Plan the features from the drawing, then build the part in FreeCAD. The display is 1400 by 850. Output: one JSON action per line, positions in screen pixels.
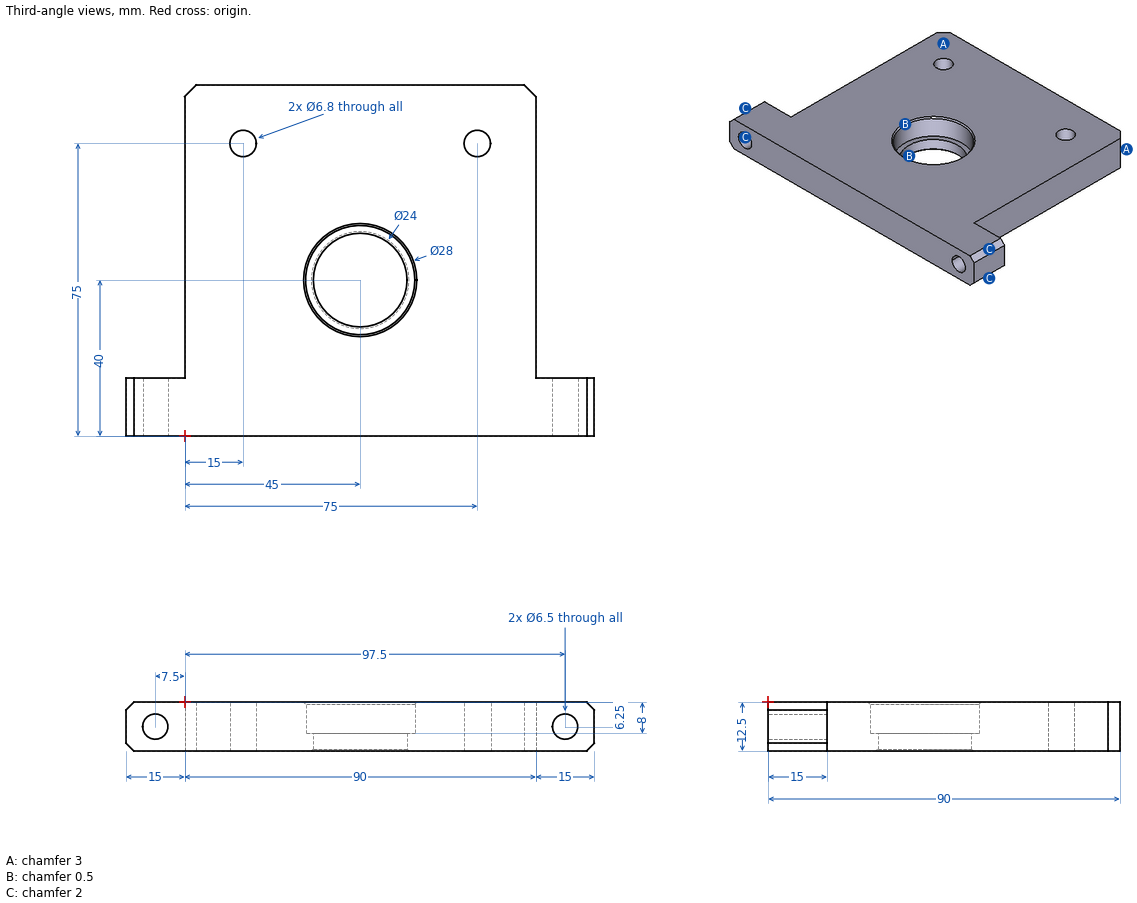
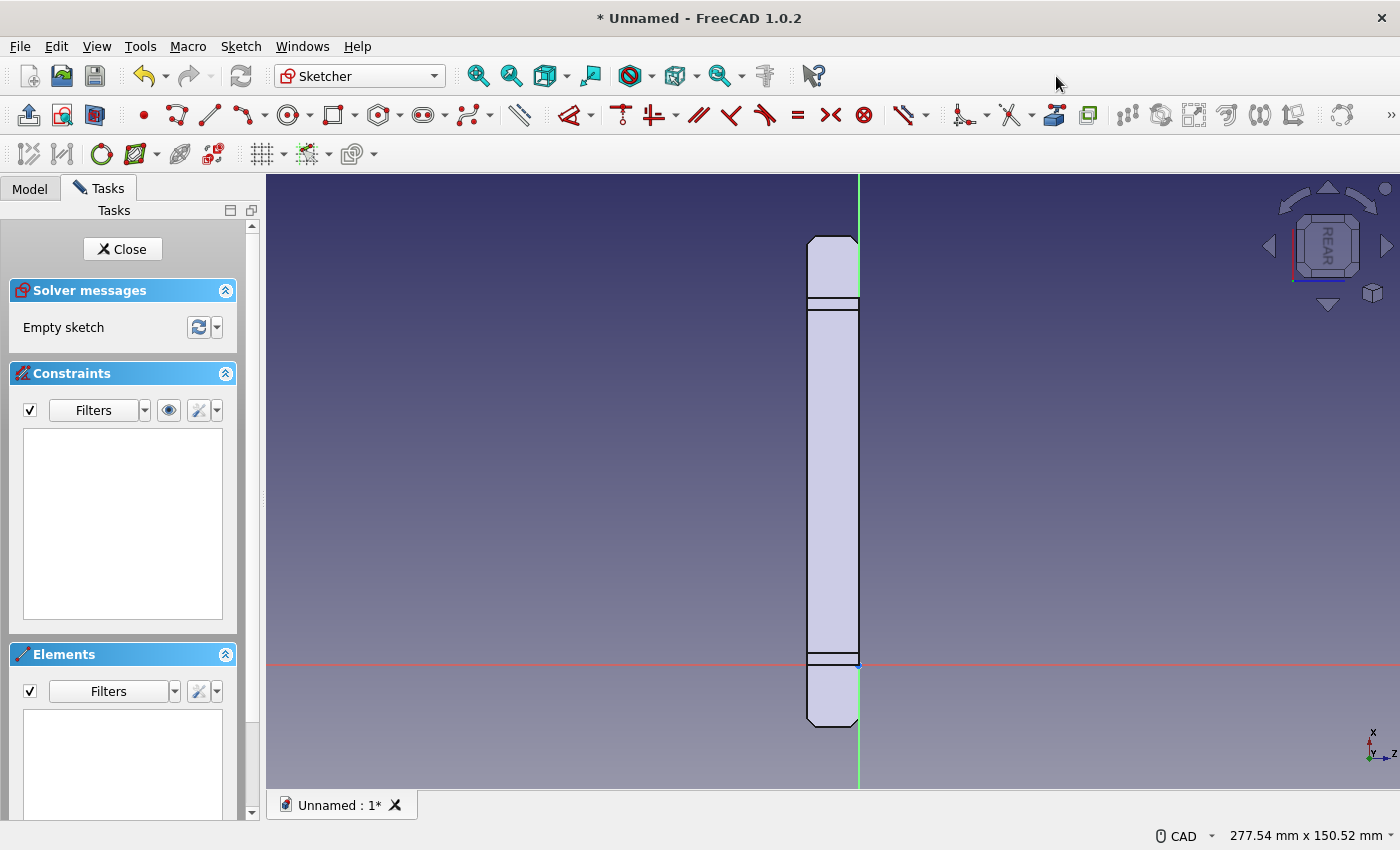
{"action": "left_click", "coordinate": [95, 116]}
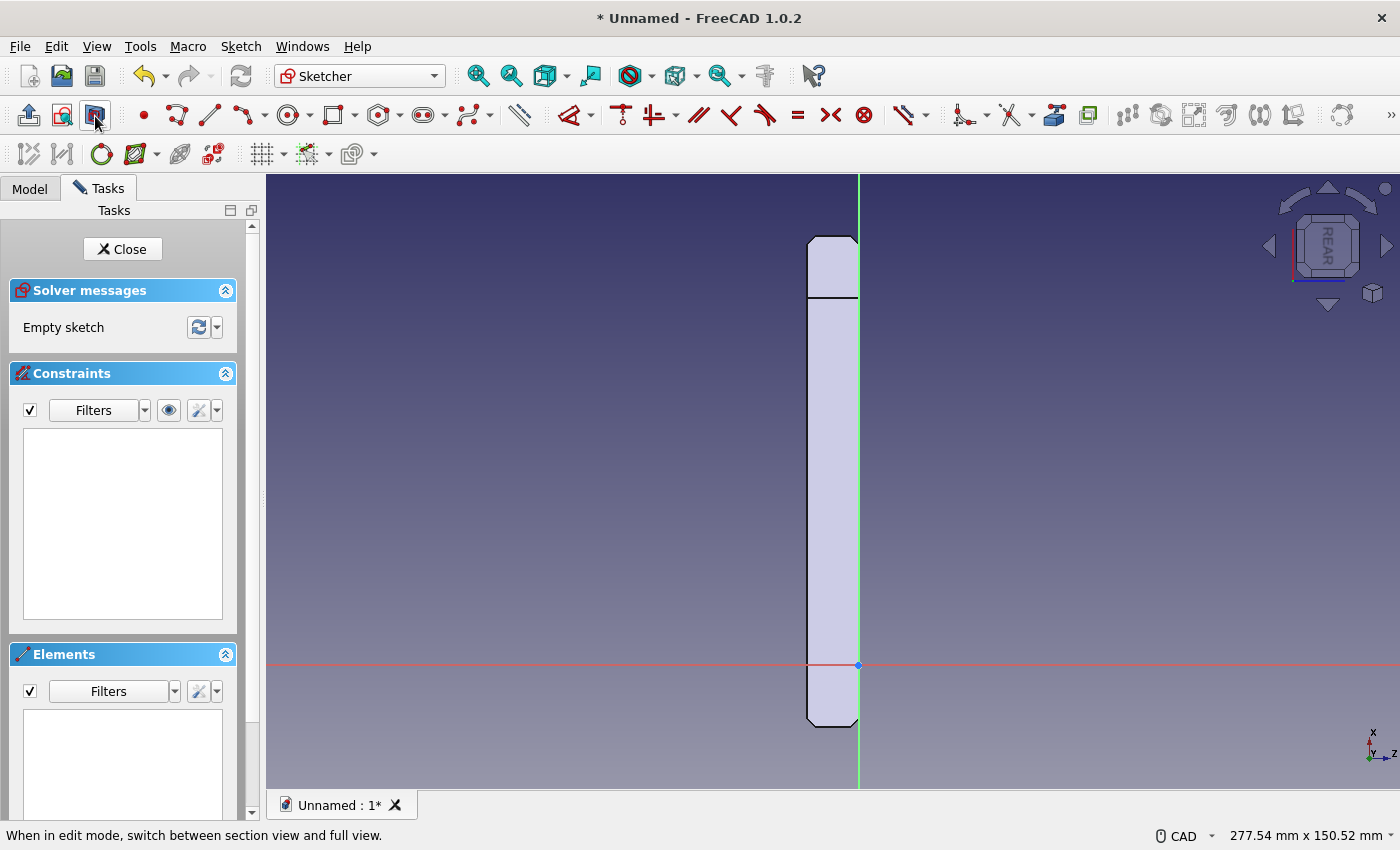
{"action": "left_click", "coordinate": [288, 116]}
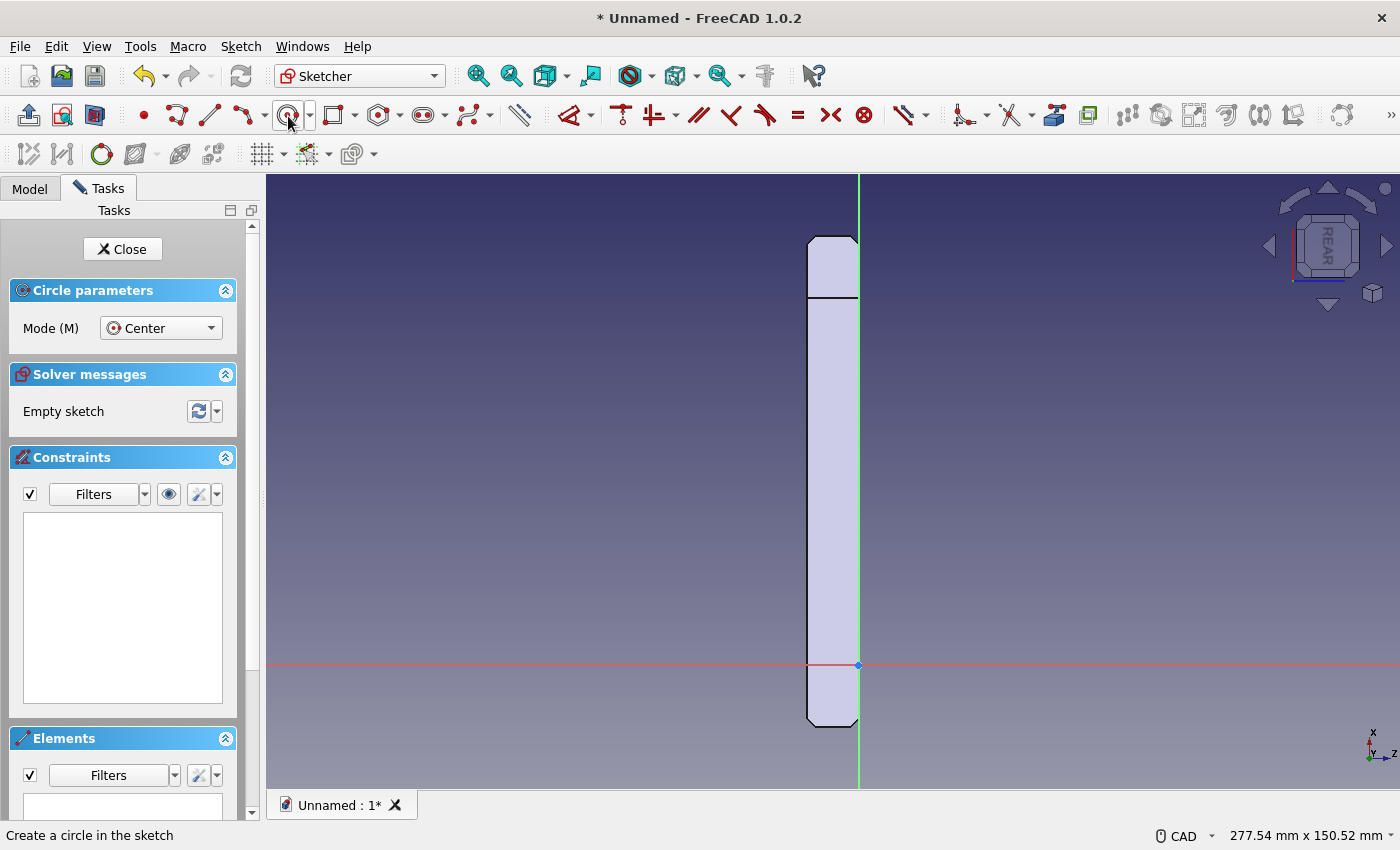
{"action": "scroll", "coordinate": [833, 267], "scroll_direction": "up", "scroll_amount": 3}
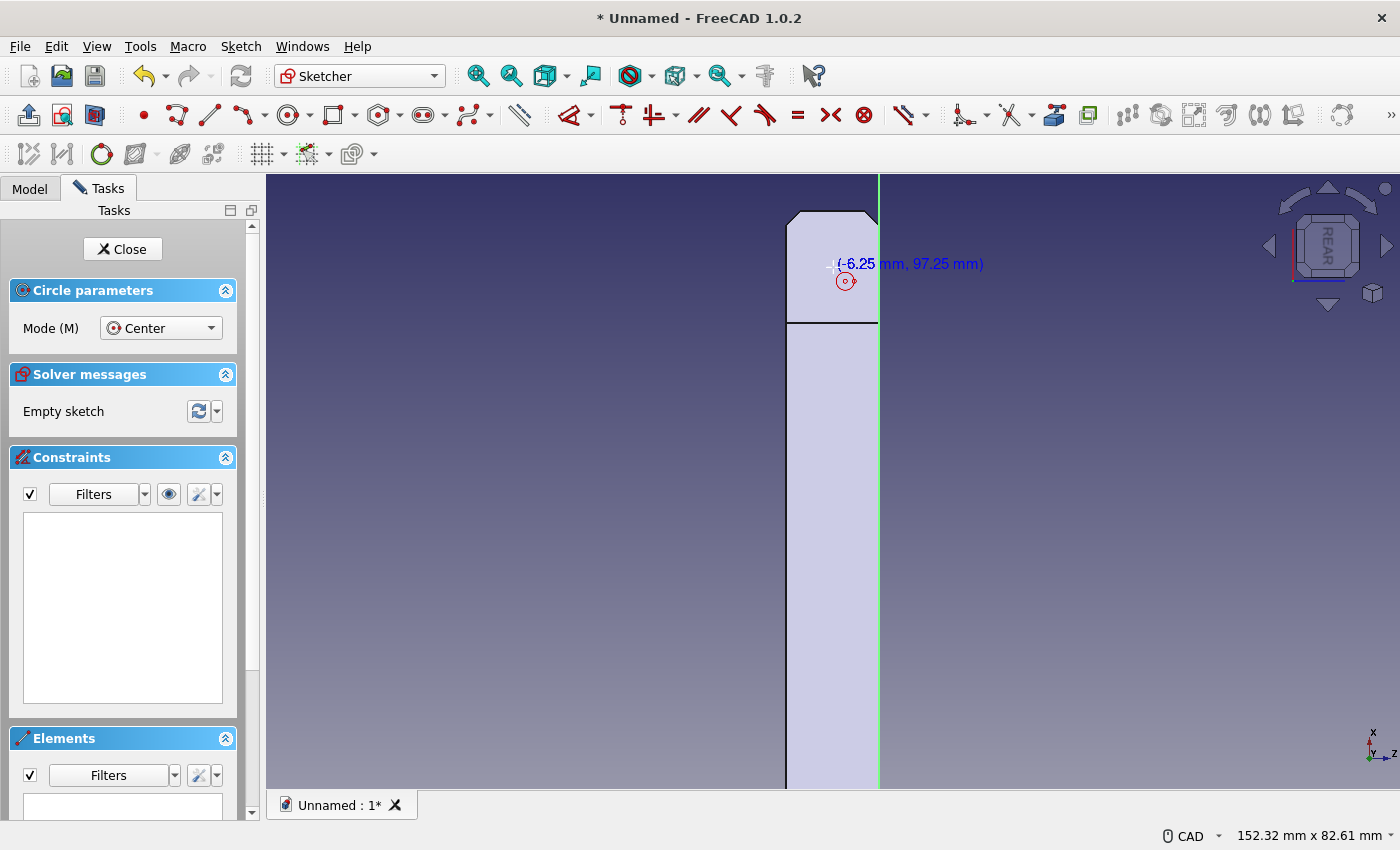
{"action": "left_click", "coordinate": [833, 267]}
{"action": "left_click", "coordinate": [850, 250]}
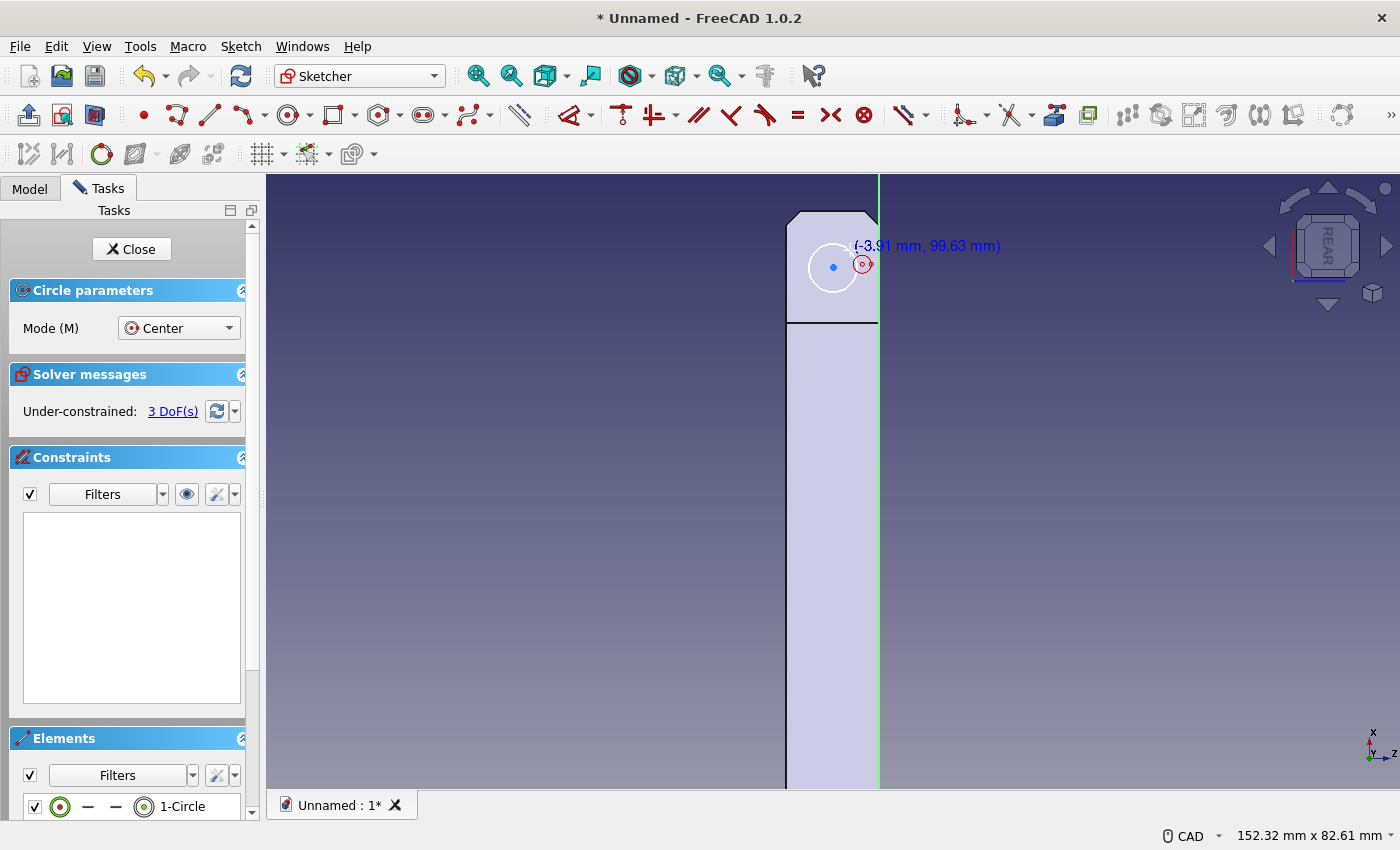
{"action": "scroll", "coordinate": [700, 338], "scroll_direction": "down", "scroll_amount": 4}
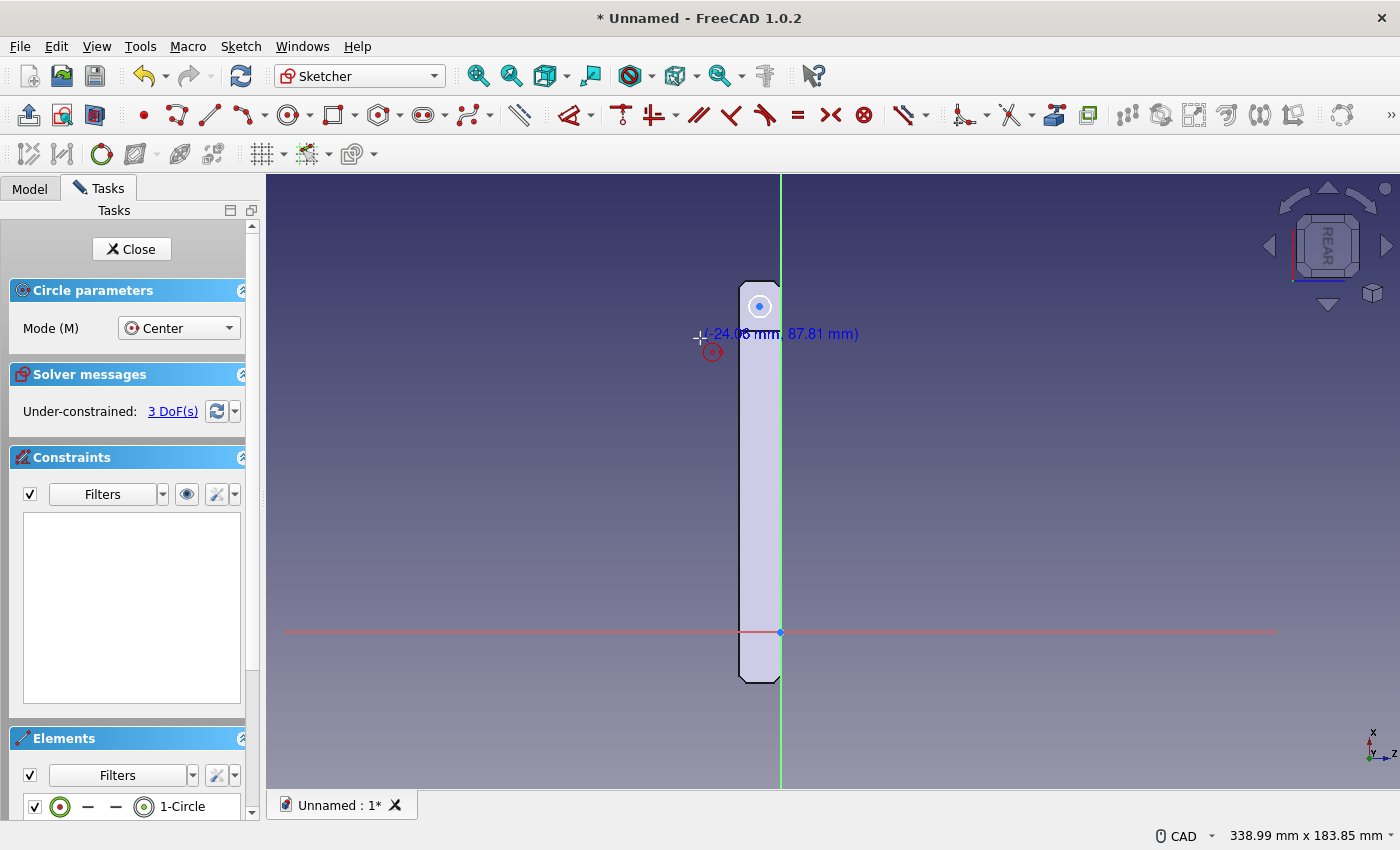
{"action": "scroll", "coordinate": [760, 657], "scroll_direction": "up", "scroll_amount": 4}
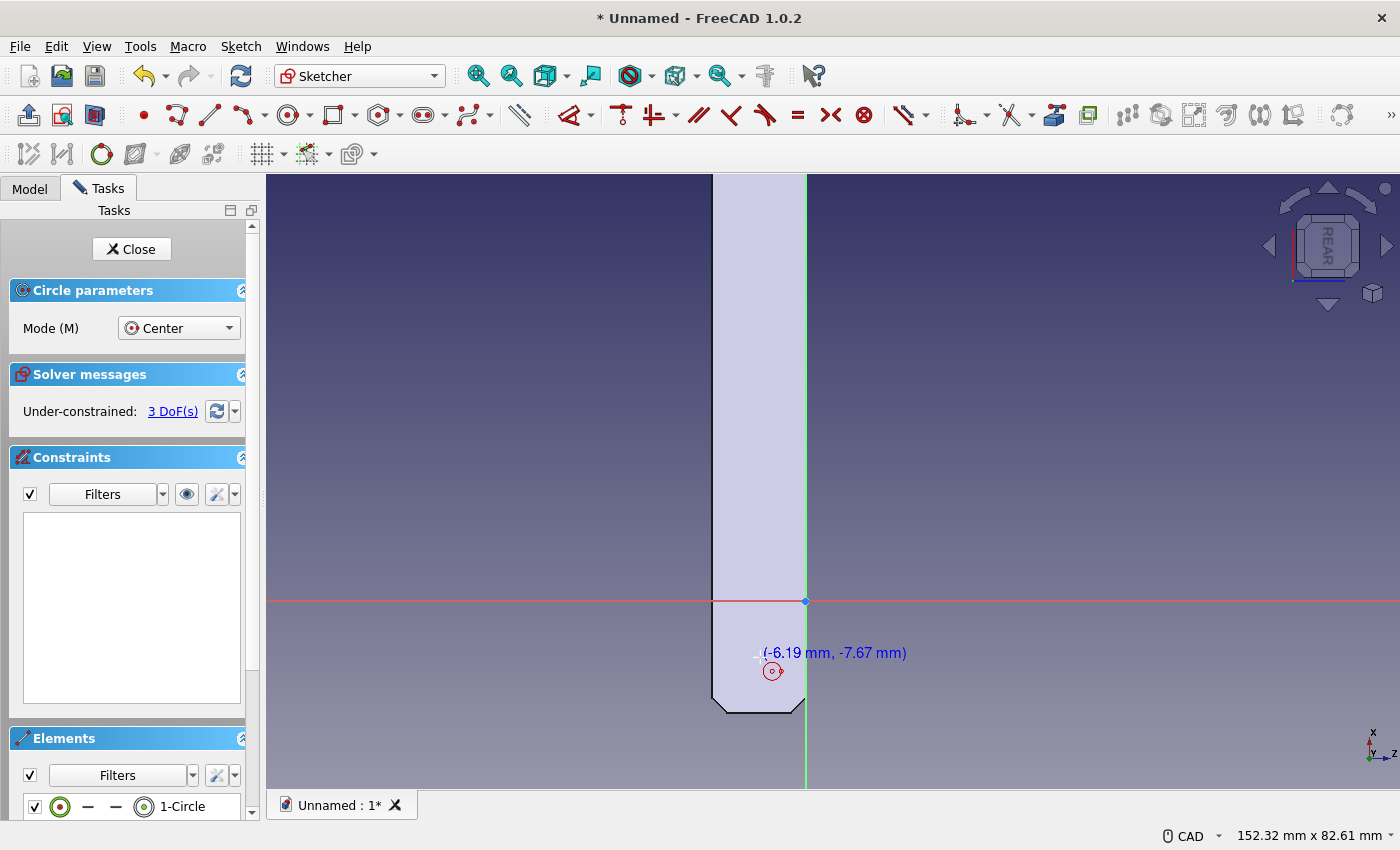
{"action": "left_click", "coordinate": [759, 657]}
{"action": "left_click", "coordinate": [776, 640]}
{"action": "key", "text": "Escape"}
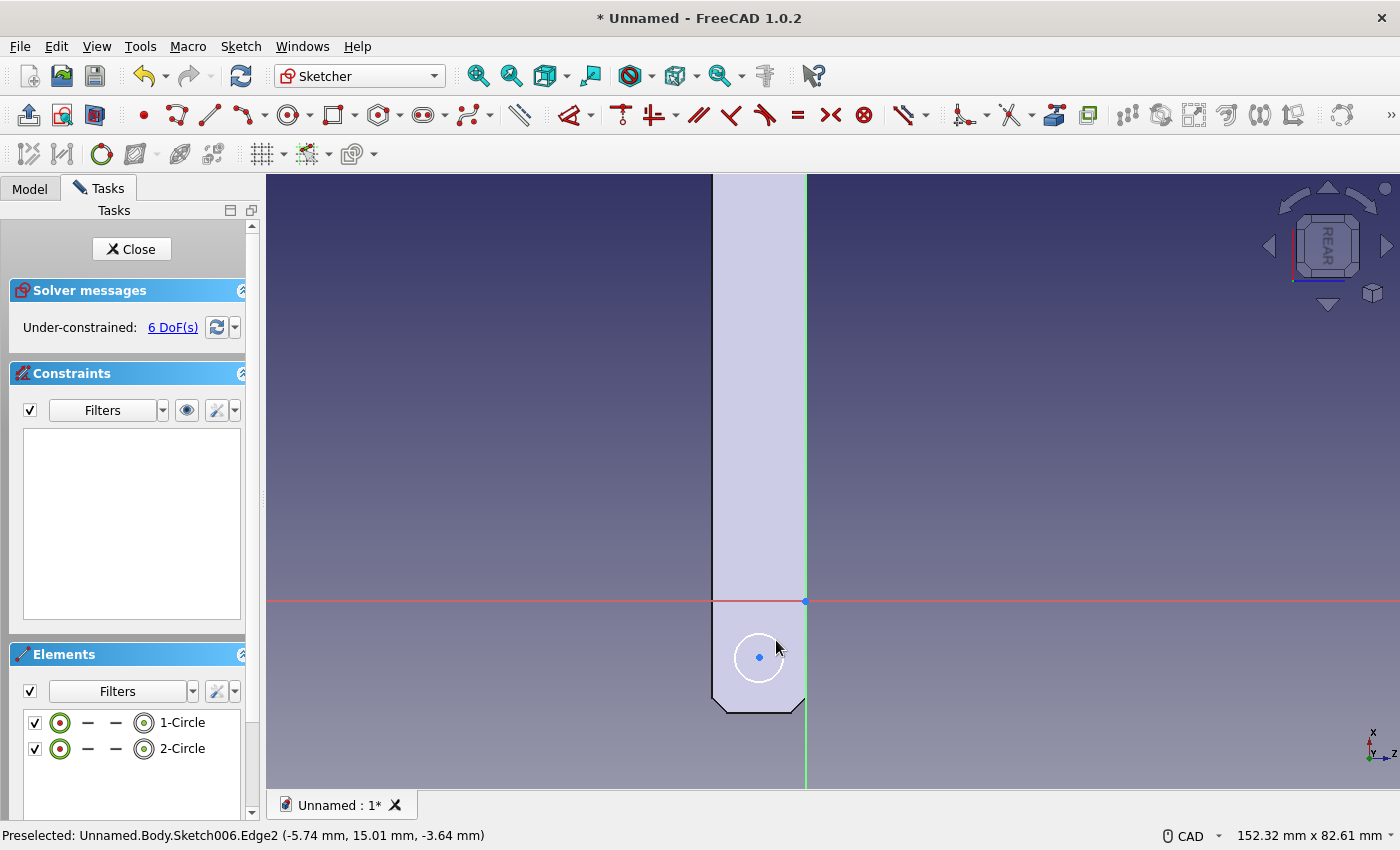
{"action": "scroll", "coordinate": [760, 657], "scroll_direction": "down", "scroll_amount": 4}